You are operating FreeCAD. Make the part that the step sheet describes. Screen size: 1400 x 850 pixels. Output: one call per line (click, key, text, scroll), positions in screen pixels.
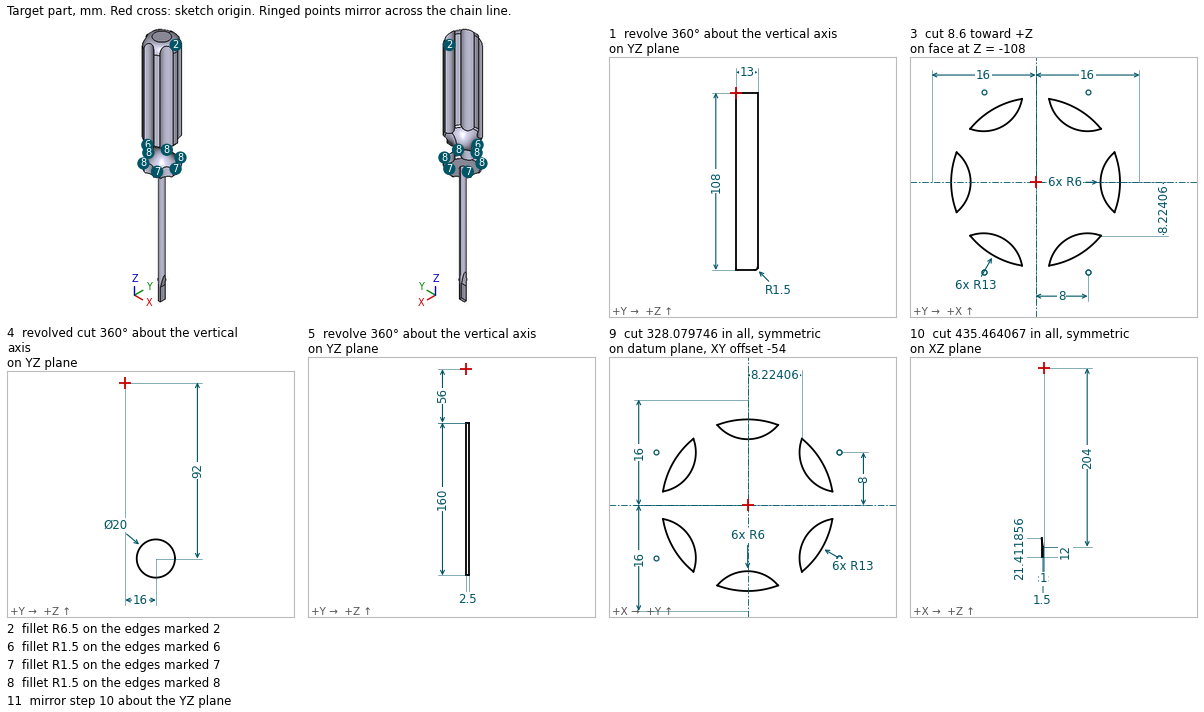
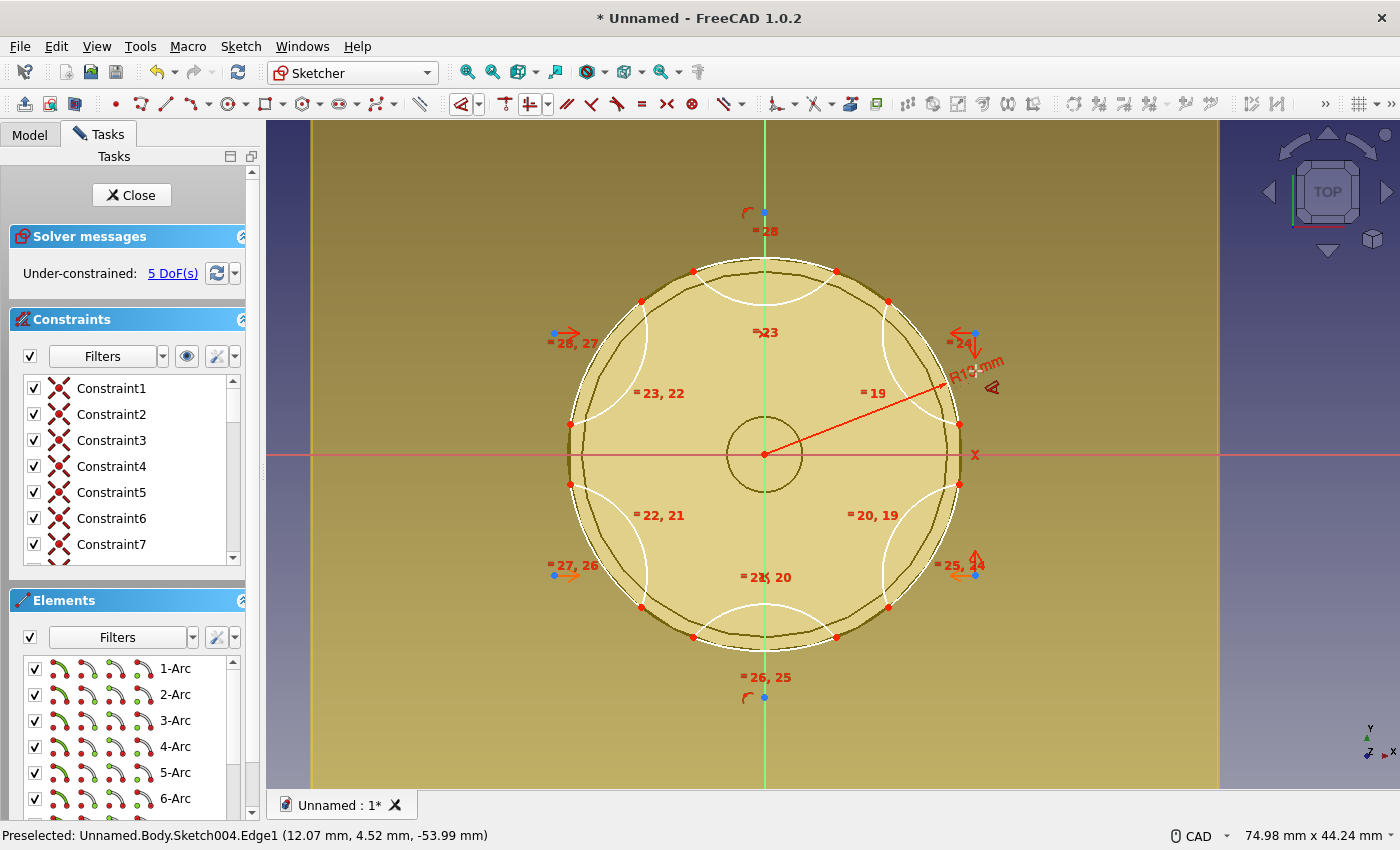
click(884, 349)
click(852, 354)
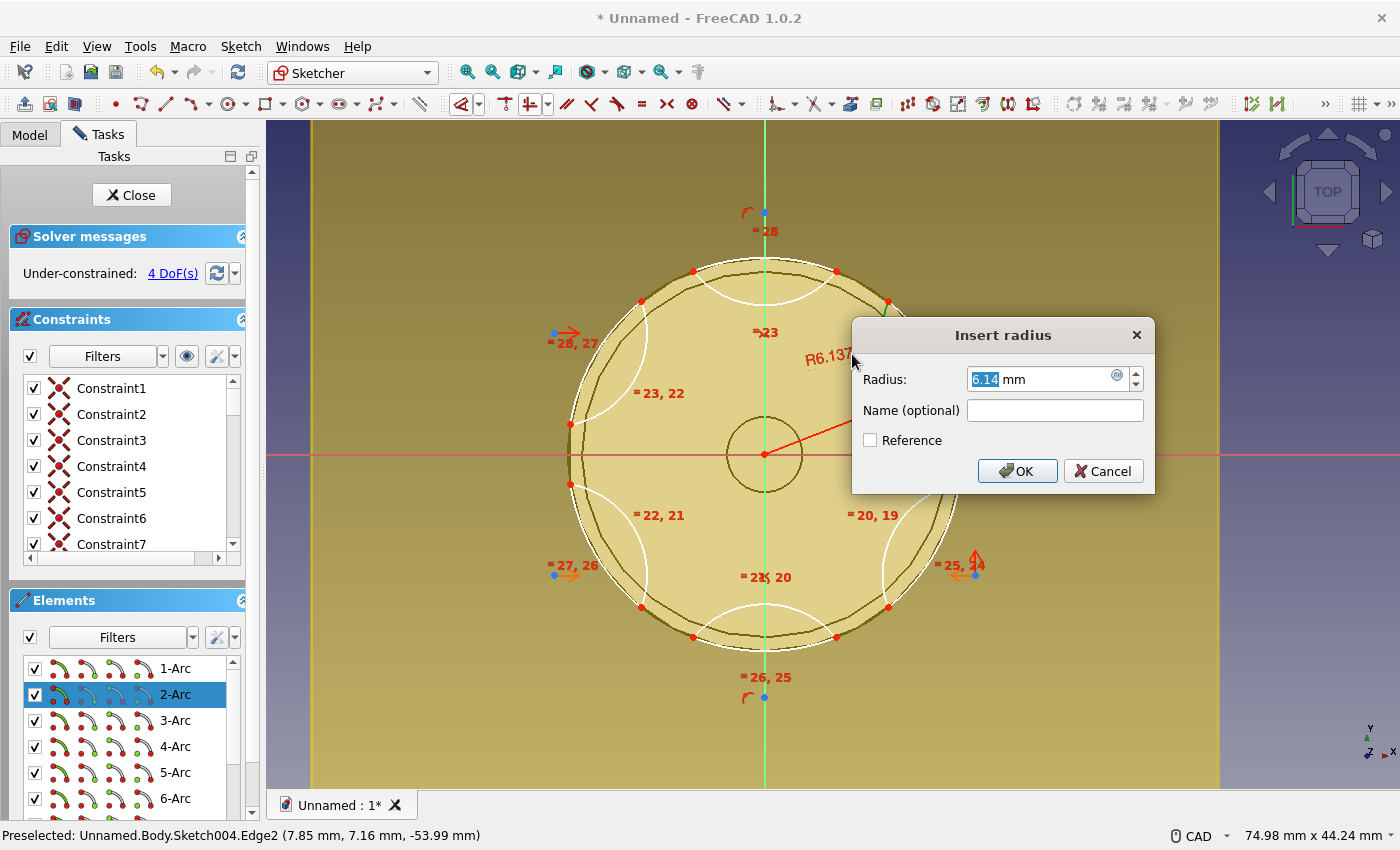
text(6)
key(Return)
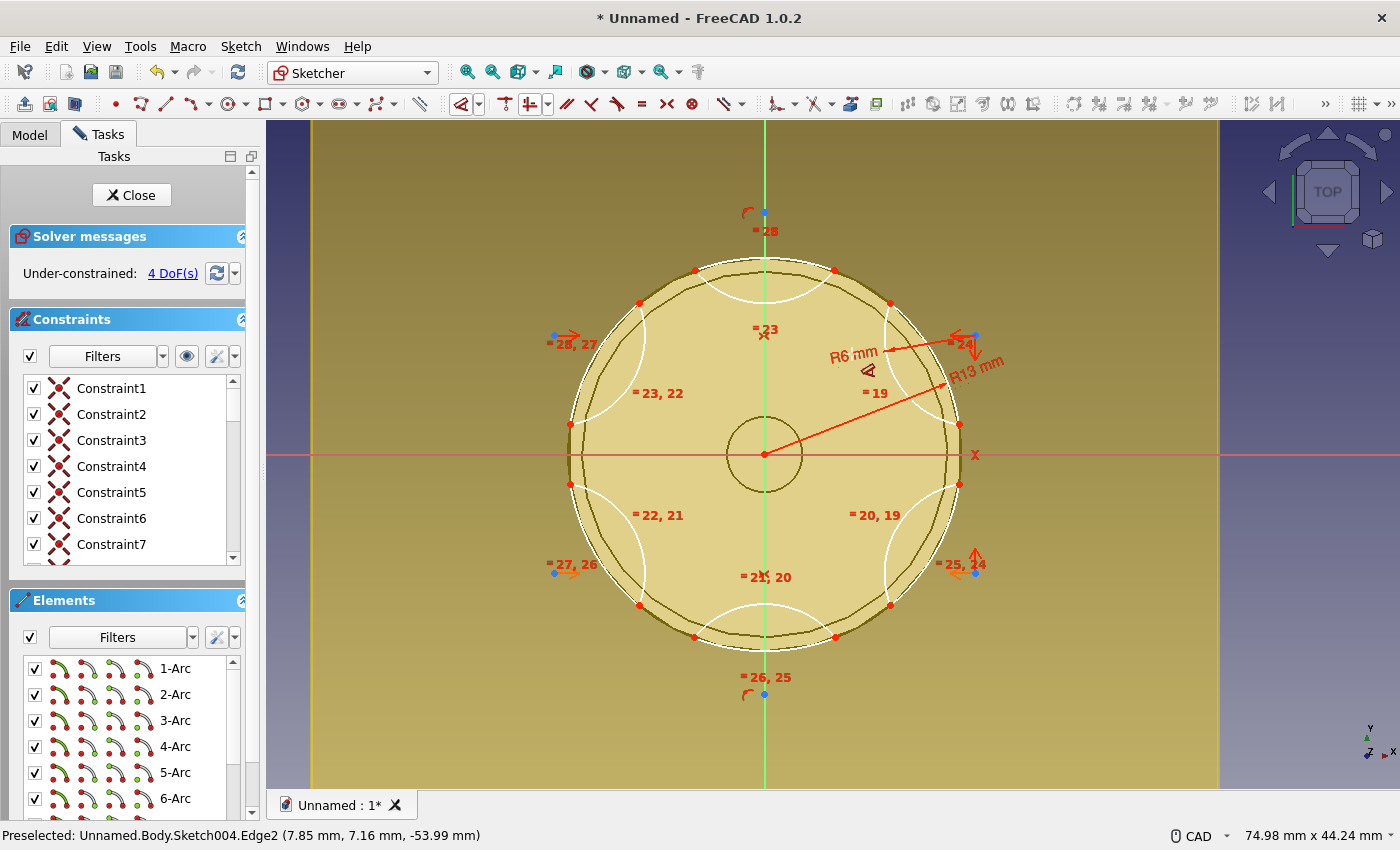
click(975, 336)
click(1009, 395)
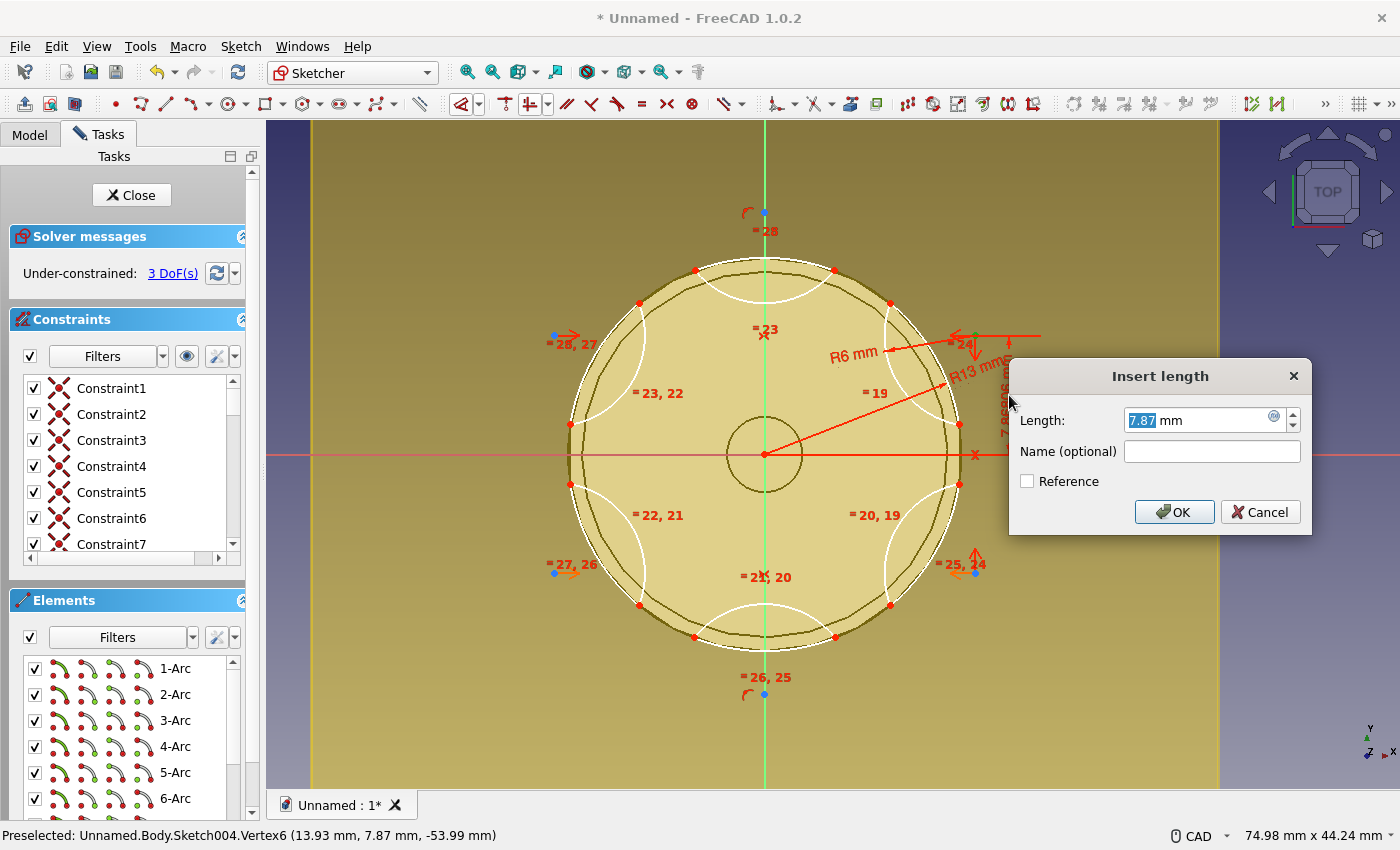
text(8)
key(Return)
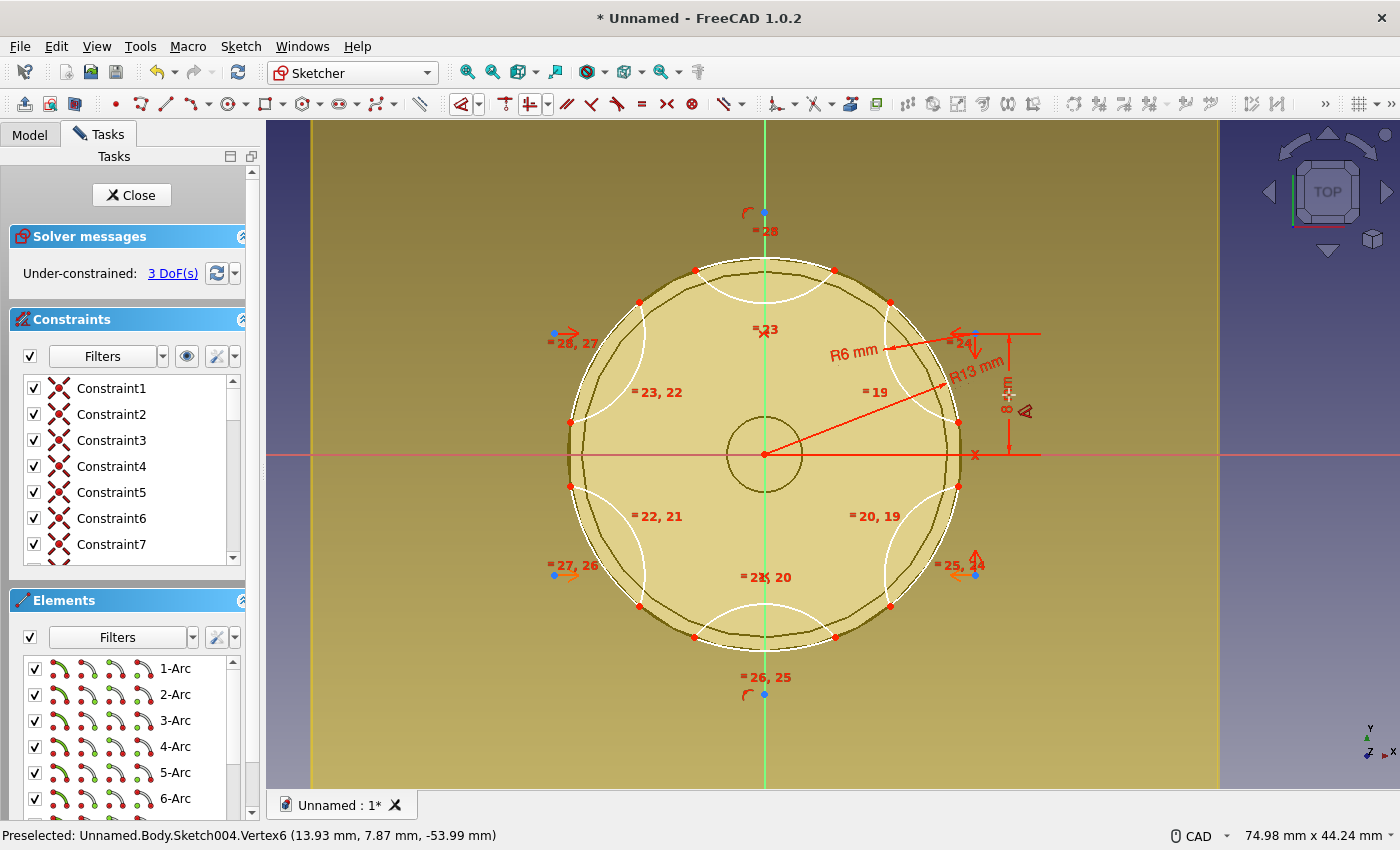
click(765, 695)
click(799, 575)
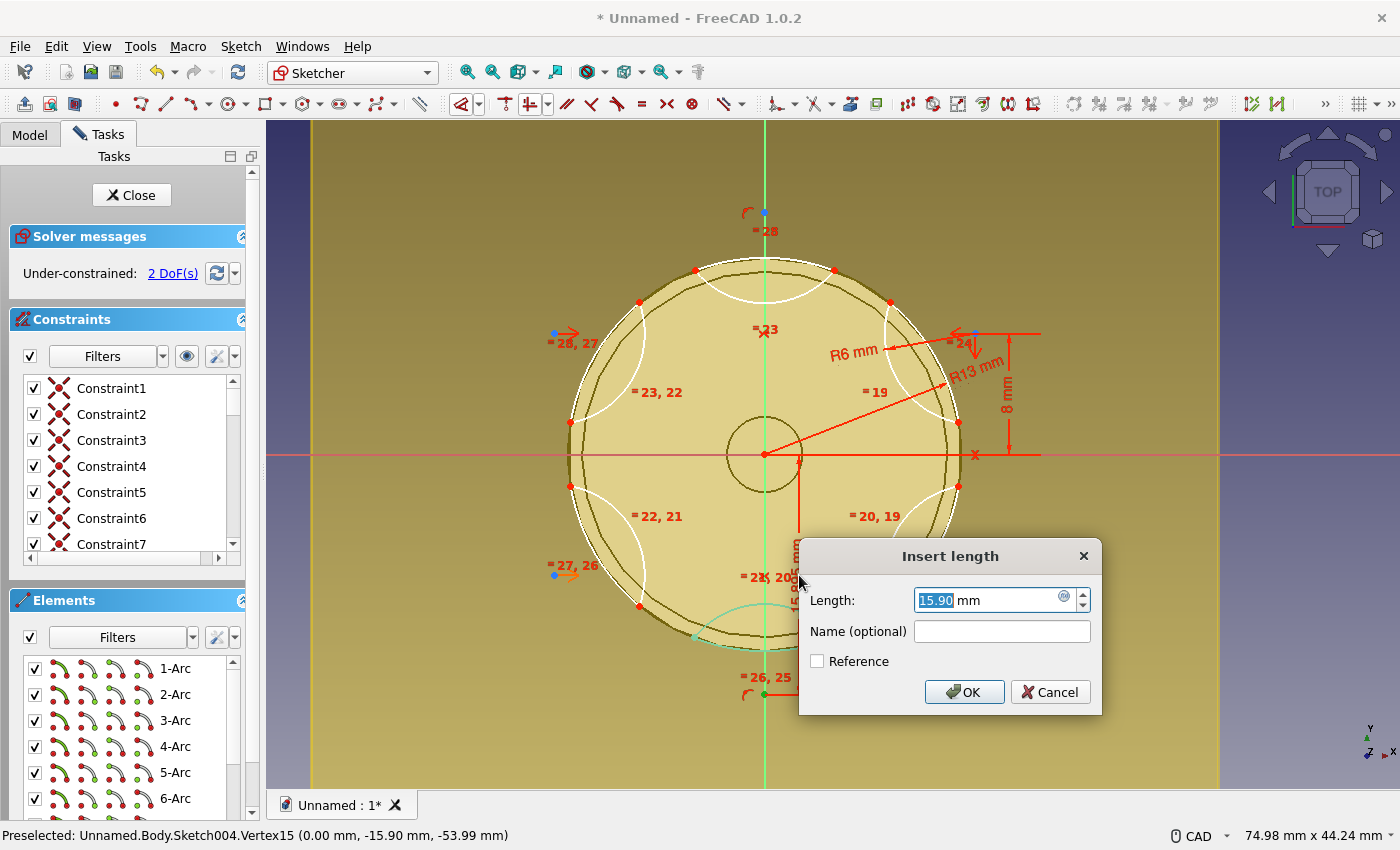
text(16)
key(Return)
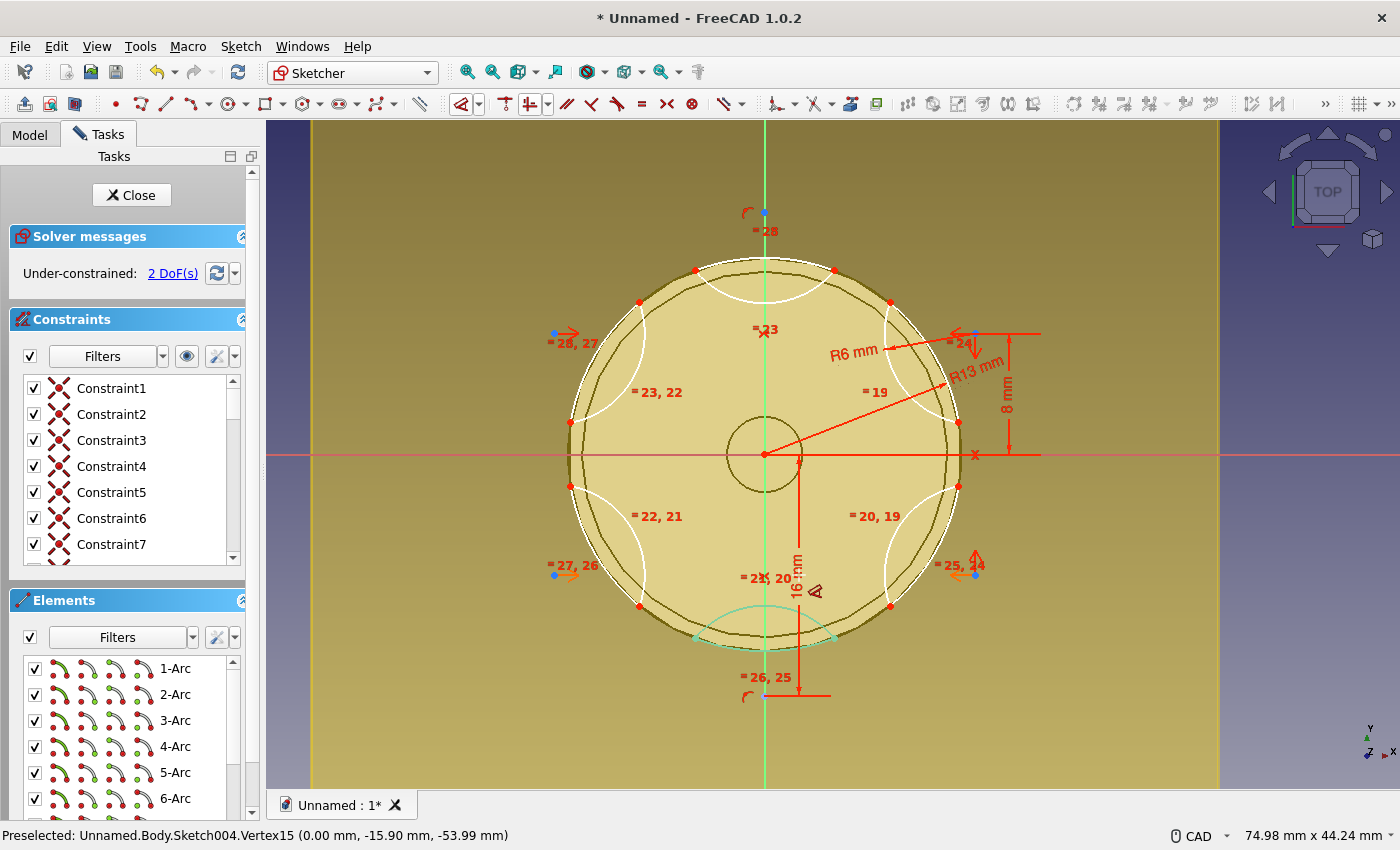
click(765, 212)
click(799, 333)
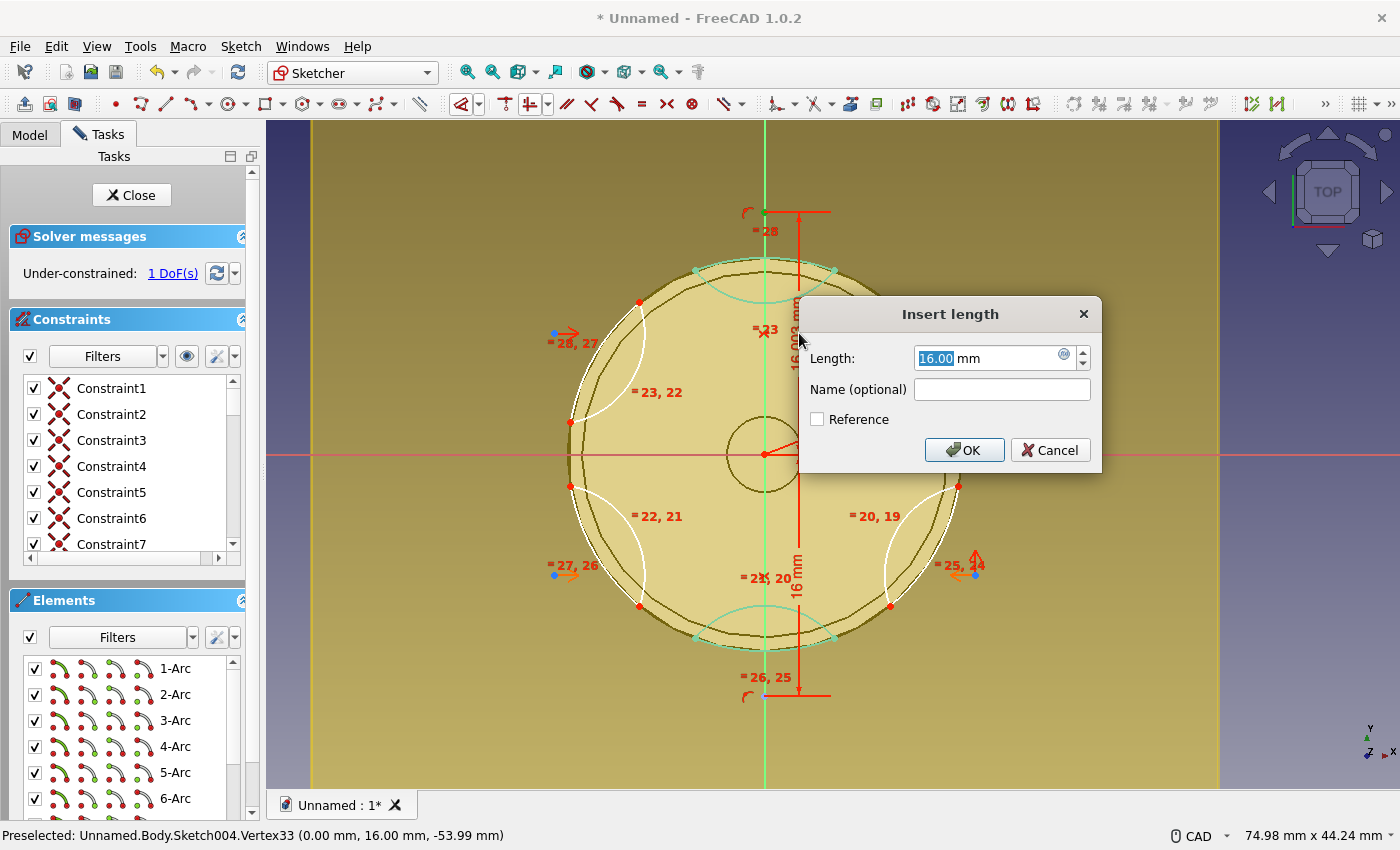
text(16)
key(Return)